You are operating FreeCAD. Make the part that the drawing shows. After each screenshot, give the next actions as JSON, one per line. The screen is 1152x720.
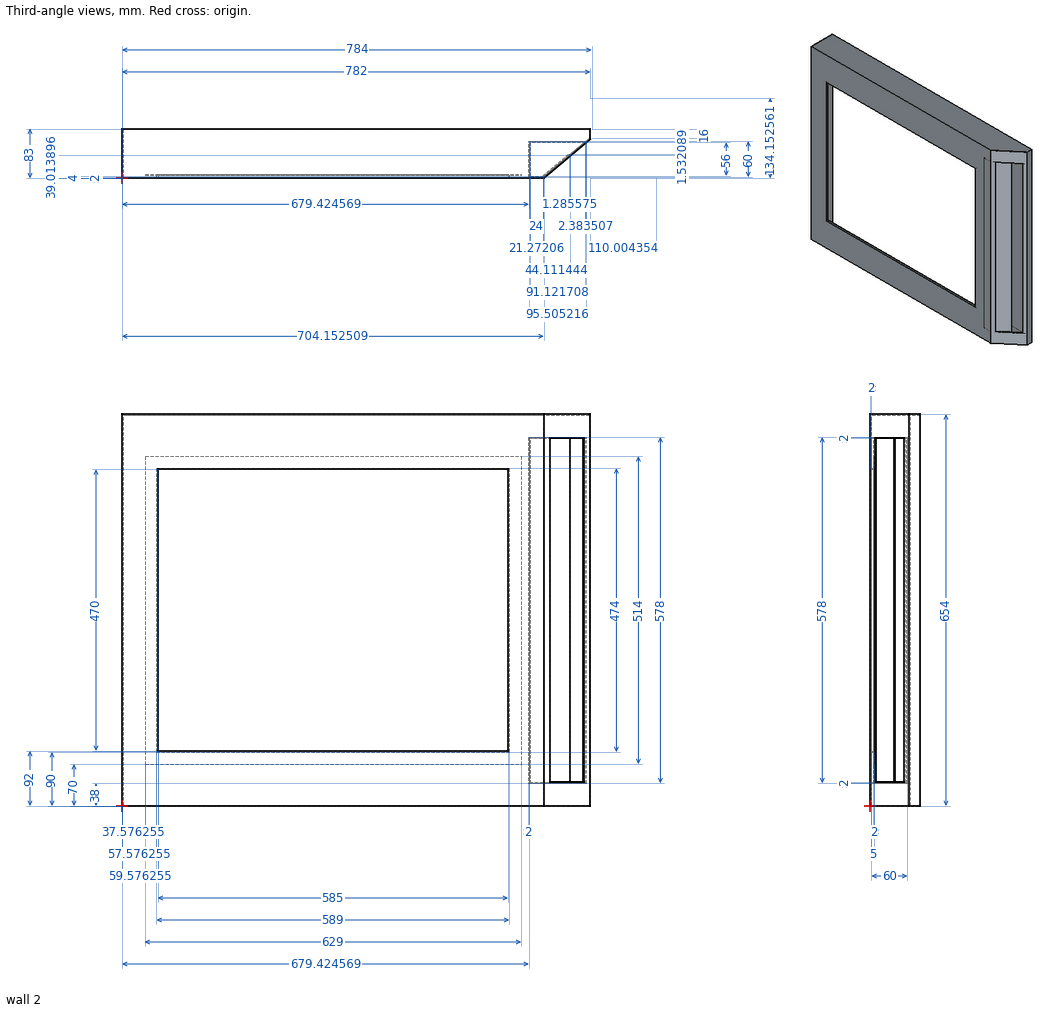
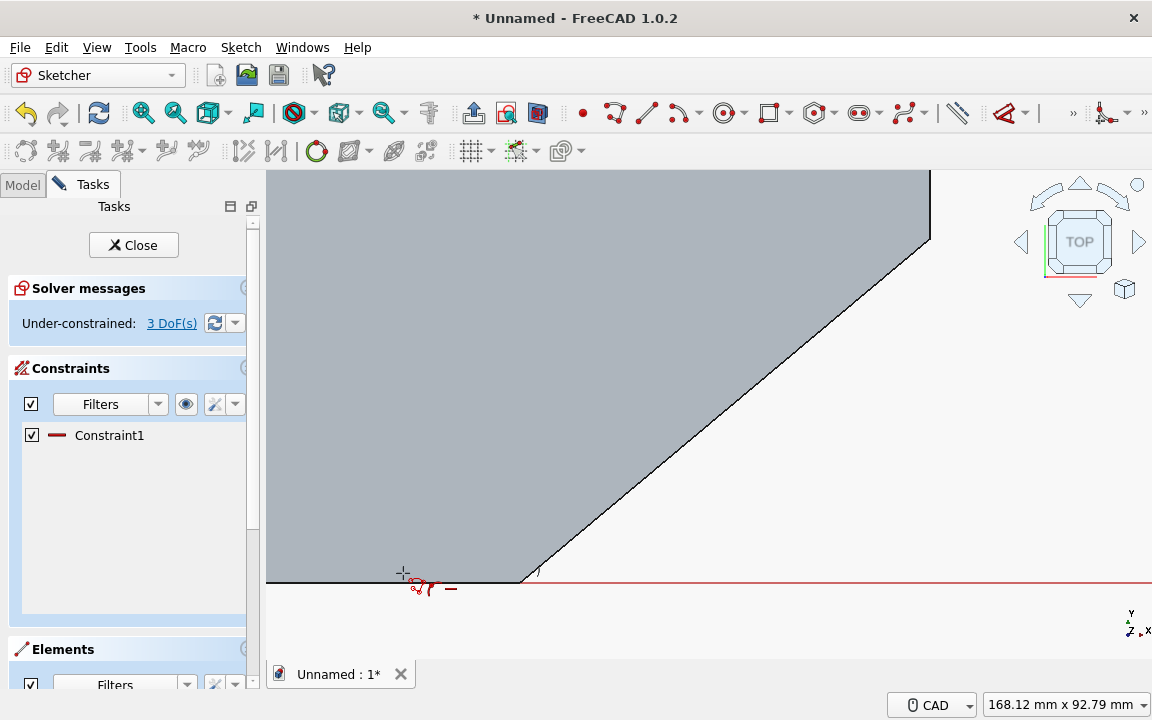
{"action": "left_click", "coordinate": [748, 378]}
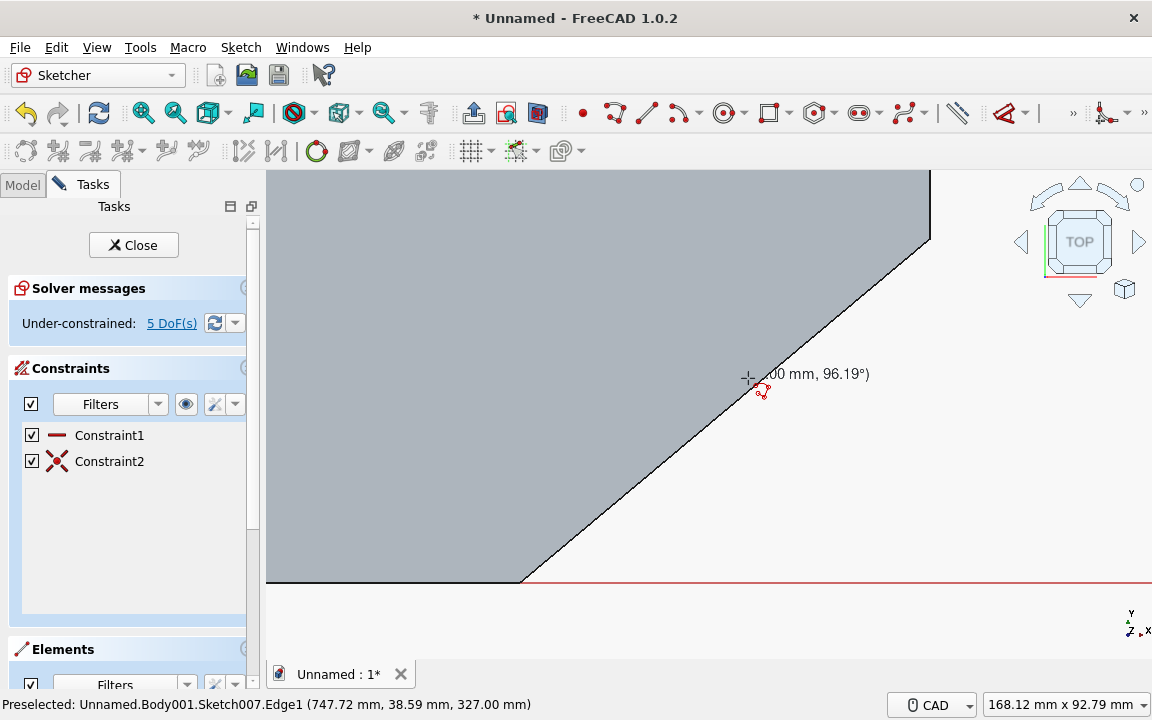
{"action": "scroll", "coordinate": [741, 370], "scroll_direction": "up", "scroll_amount": 3}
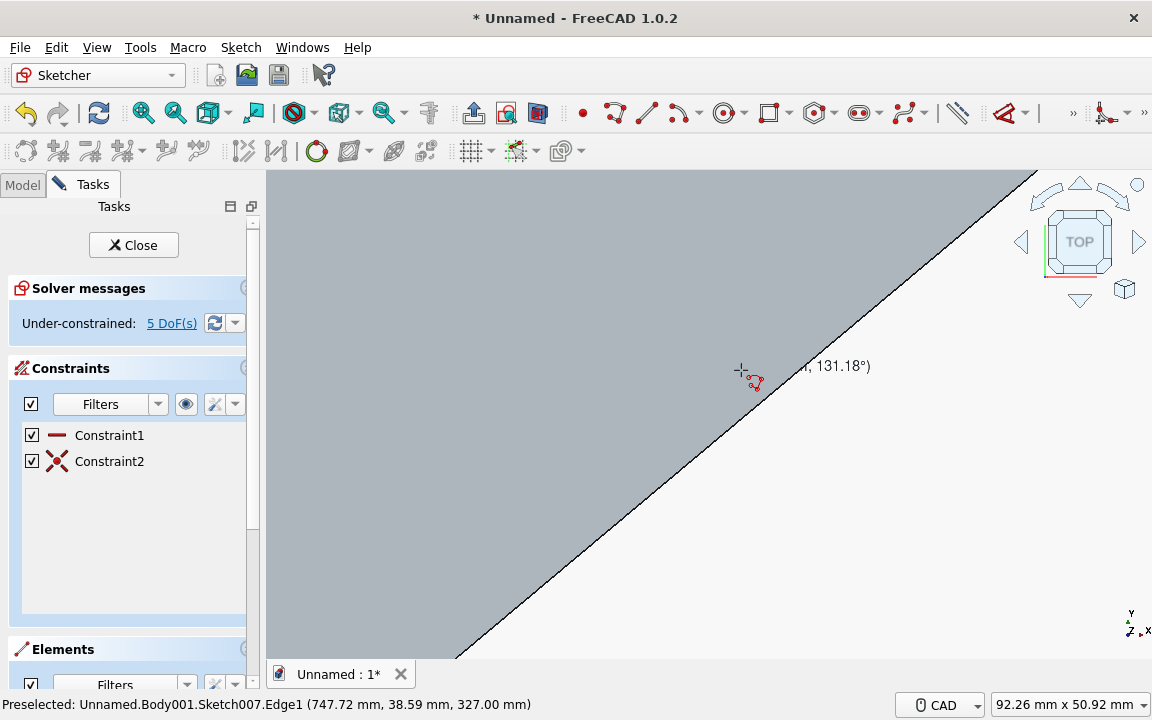
{"action": "left_click", "coordinate": [741, 369]}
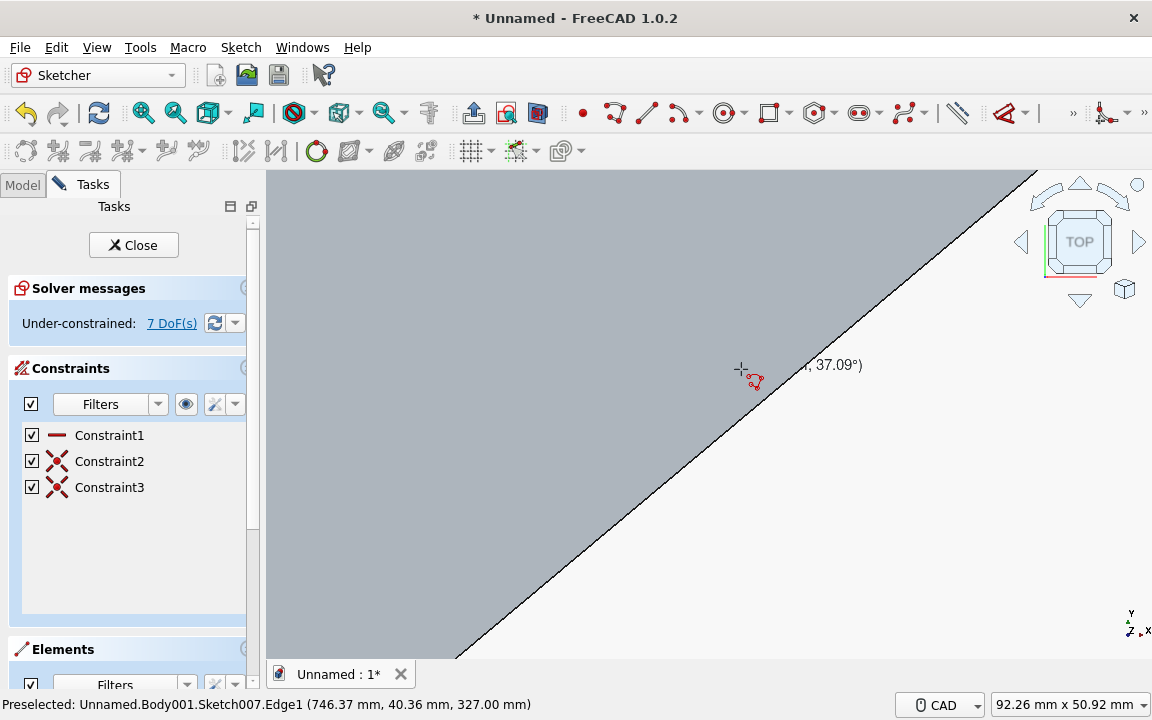
{"action": "scroll", "coordinate": [741, 370], "scroll_direction": "down", "scroll_amount": 3}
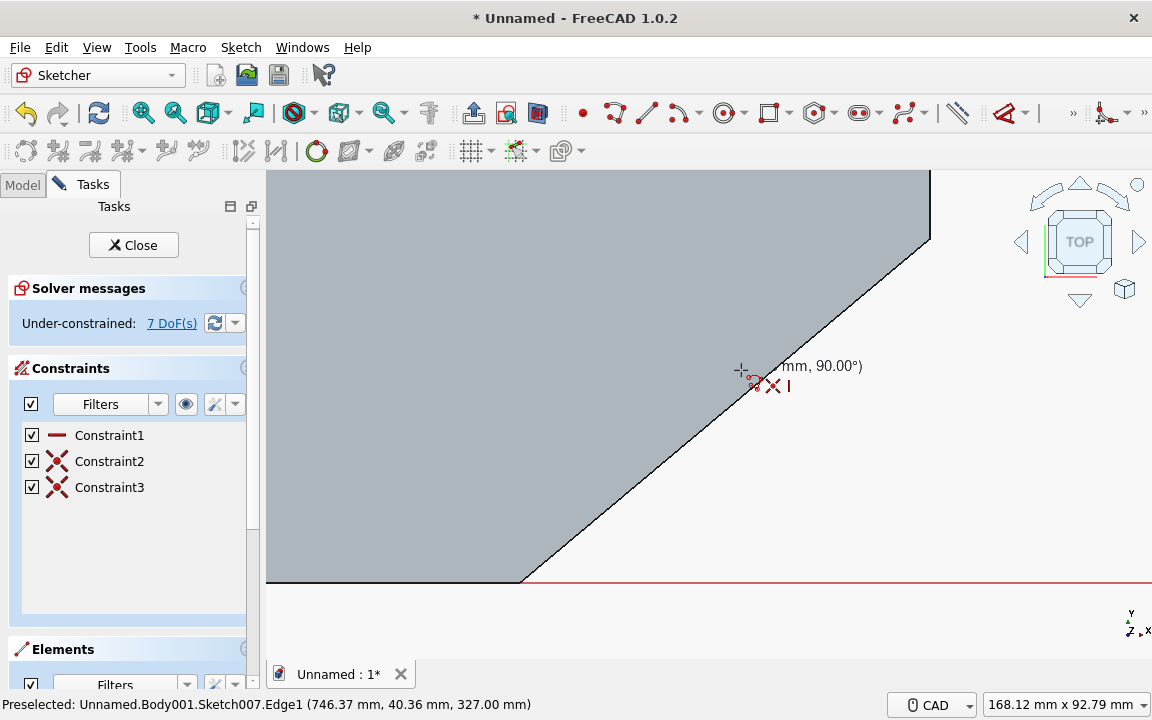
{"action": "scroll", "coordinate": [512, 562], "scroll_direction": "up", "scroll_amount": 3}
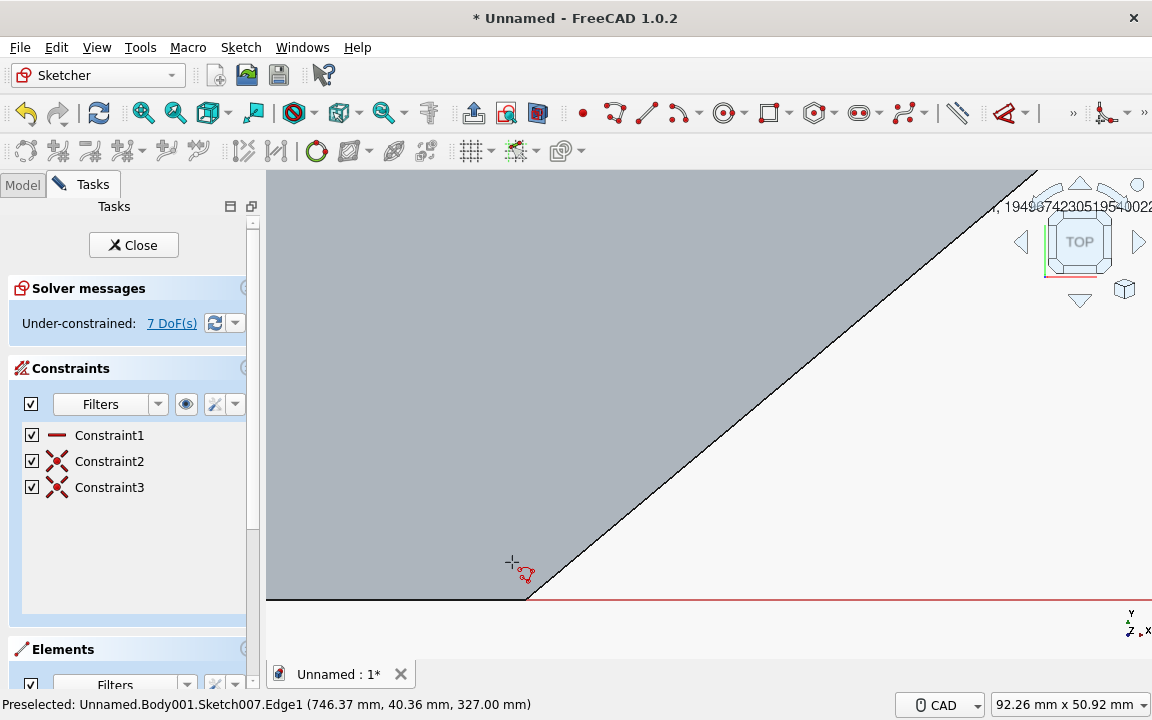
{"action": "left_click", "coordinate": [511, 562]}
{"action": "left_click", "coordinate": [307, 562]}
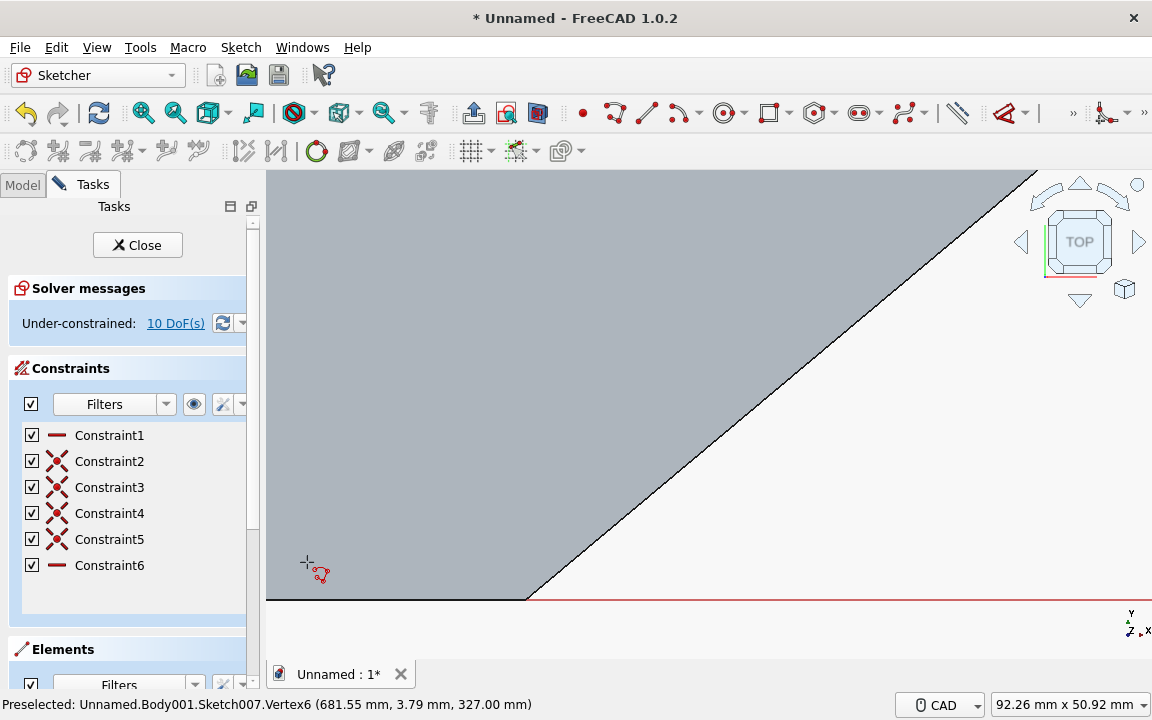
{"action": "scroll", "coordinate": [512, 562], "scroll_direction": "down", "scroll_amount": 3}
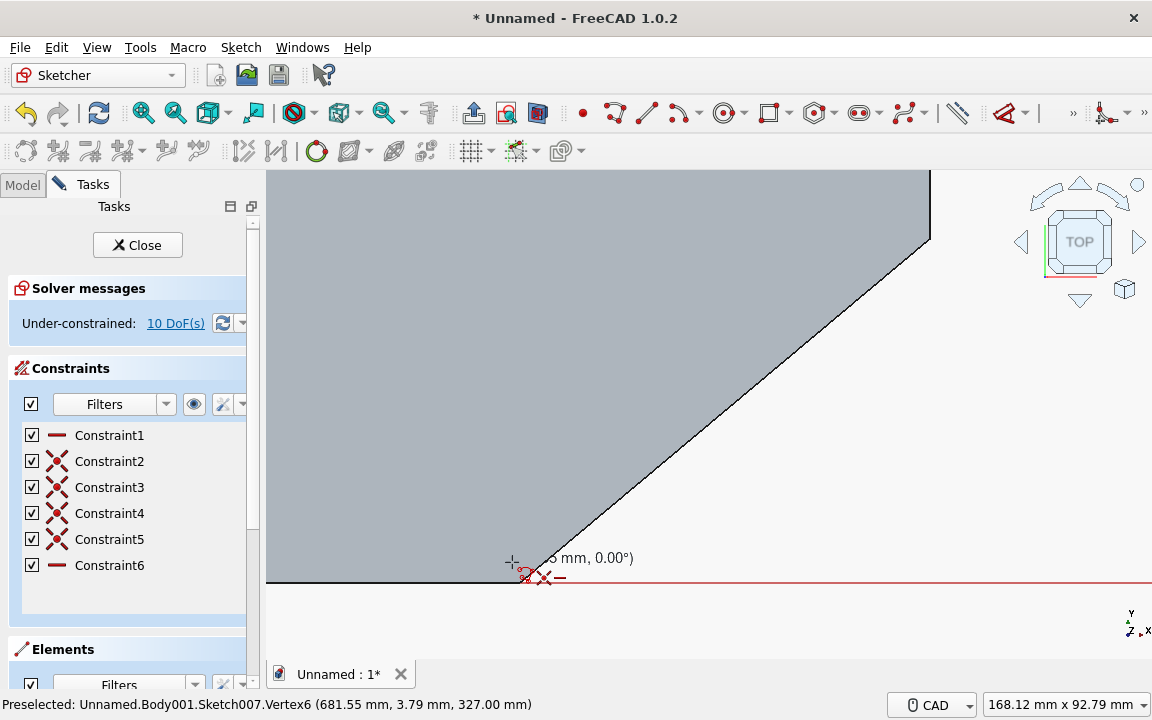
{"action": "left_click", "coordinate": [400, 267]}
{"action": "left_click", "coordinate": [880, 267]}
{"action": "left_click", "coordinate": [892, 257]}
{"action": "left_click", "coordinate": [389, 257]}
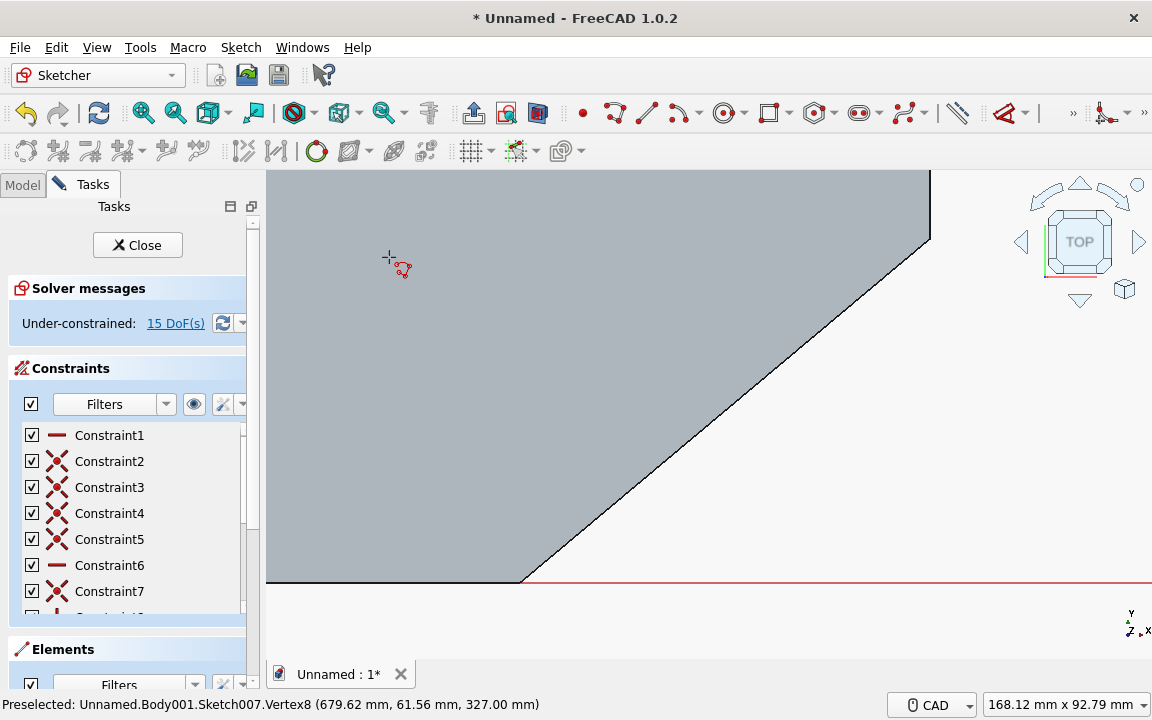
{"action": "scroll", "coordinate": [389, 573], "scroll_direction": "up", "scroll_amount": 3}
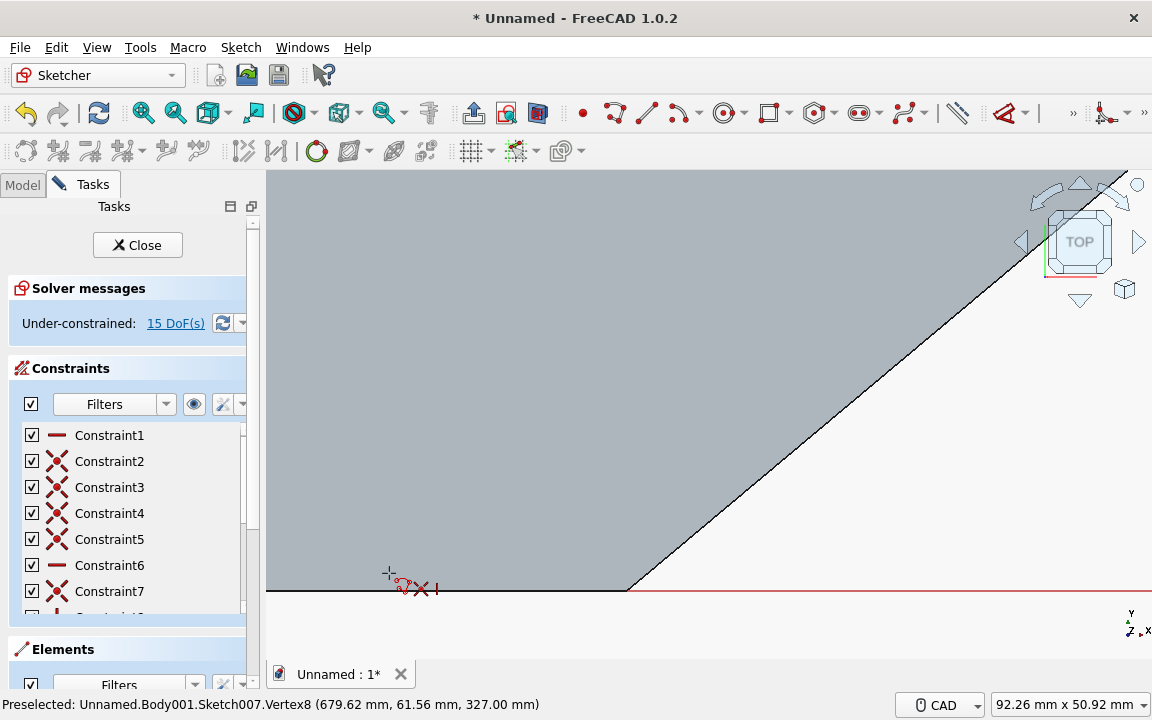
{"action": "left_click", "coordinate": [389, 573]}
{"action": "key", "text": "Escape"}
{"action": "key", "text": "Escape"}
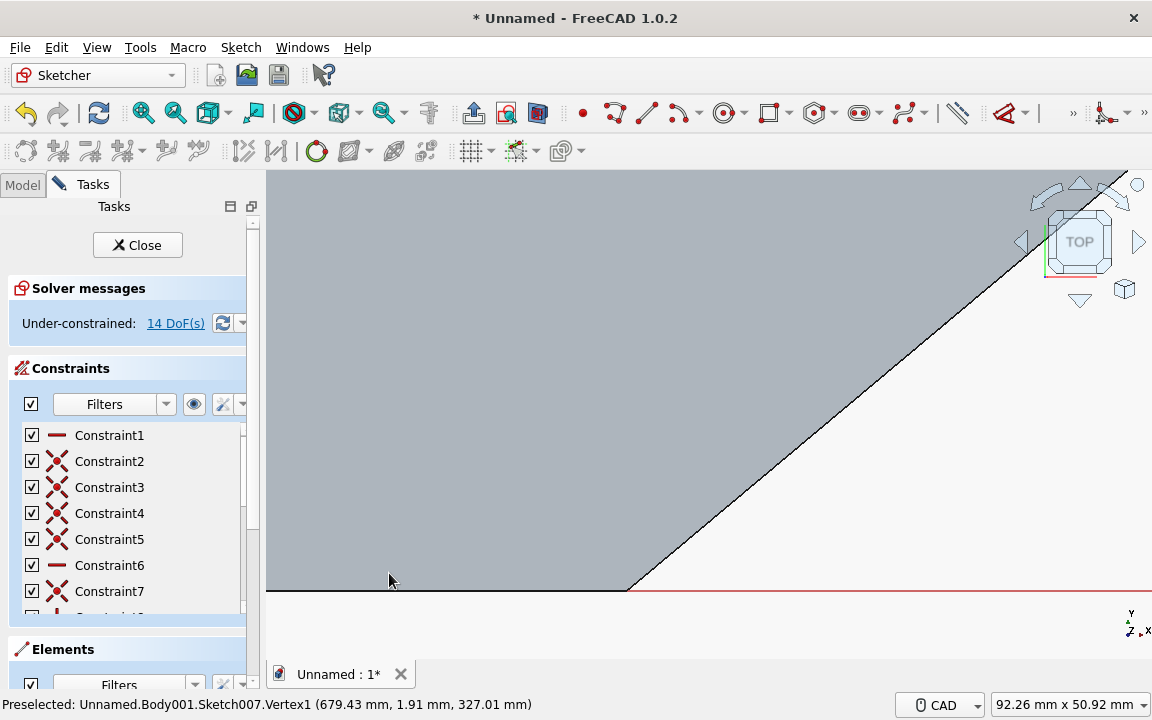
{"action": "key", "text": "d"}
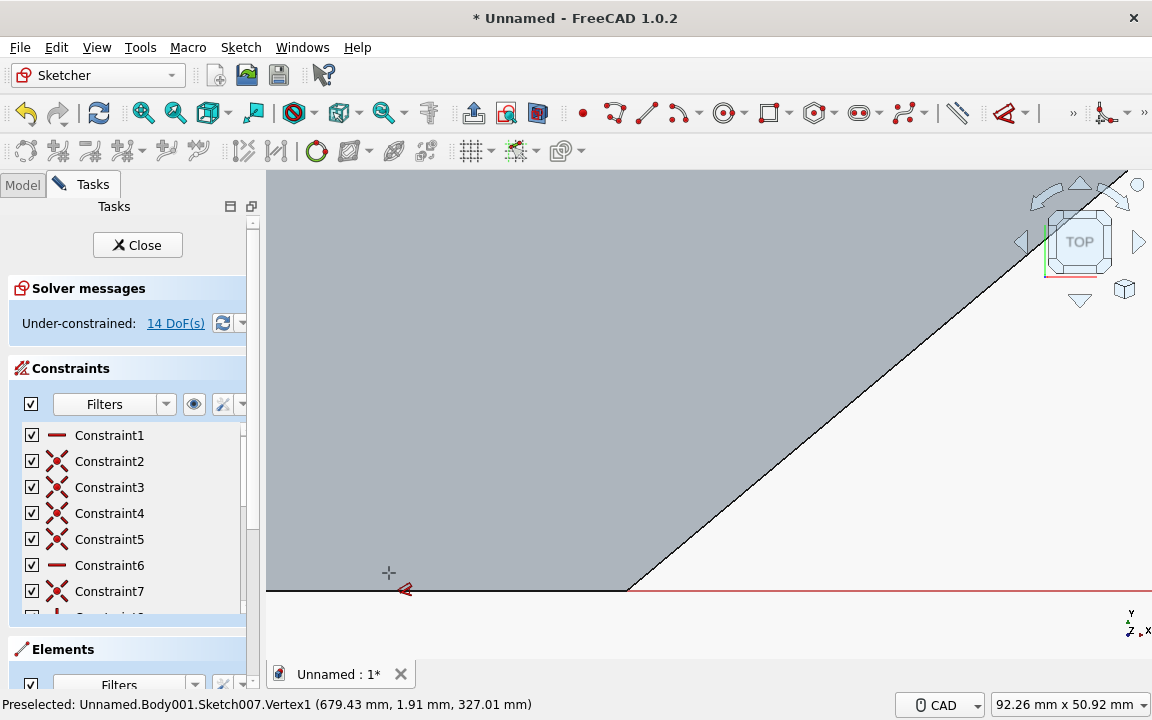
{"action": "left_click", "coordinate": [458, 573]}
{"action": "left_click", "coordinate": [504, 607]}